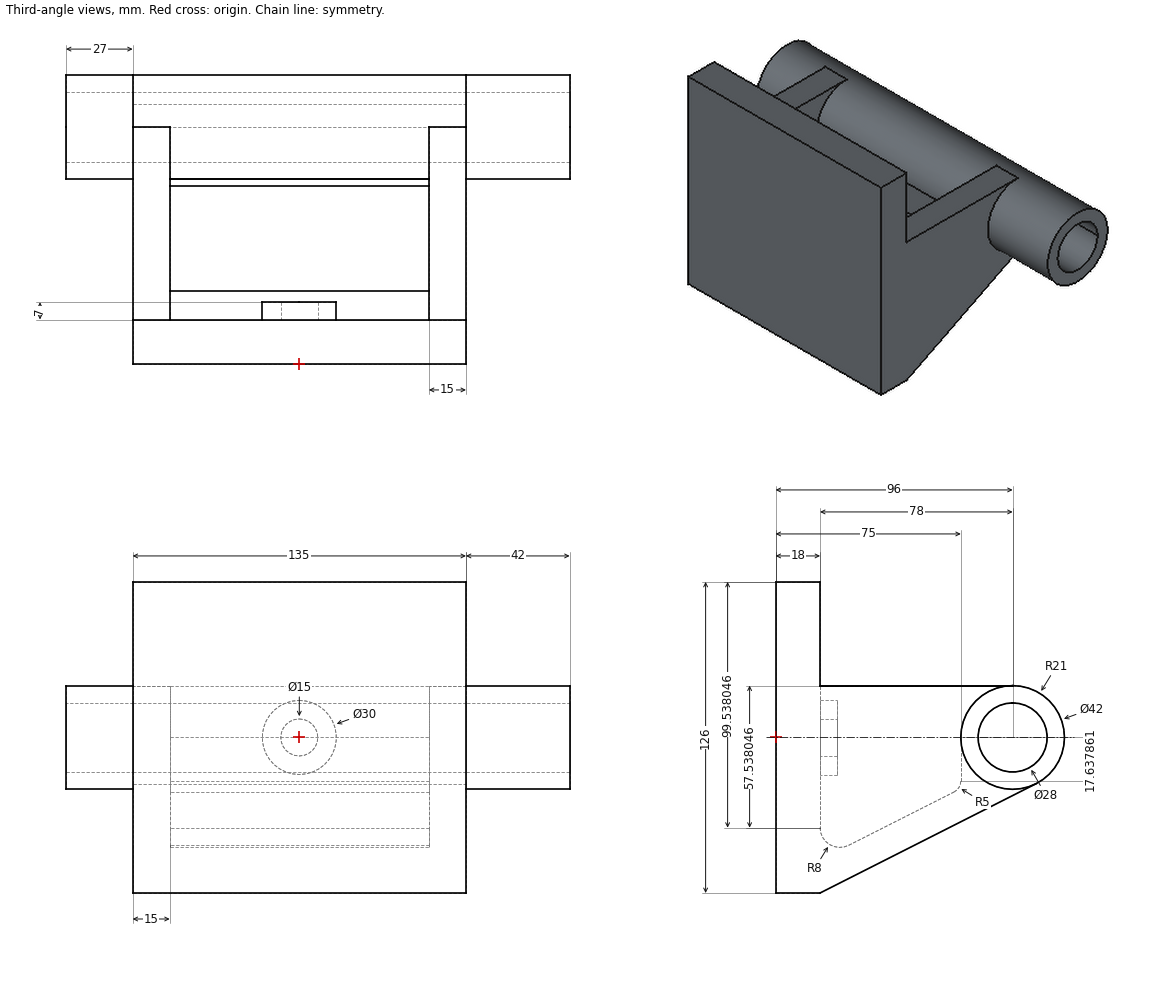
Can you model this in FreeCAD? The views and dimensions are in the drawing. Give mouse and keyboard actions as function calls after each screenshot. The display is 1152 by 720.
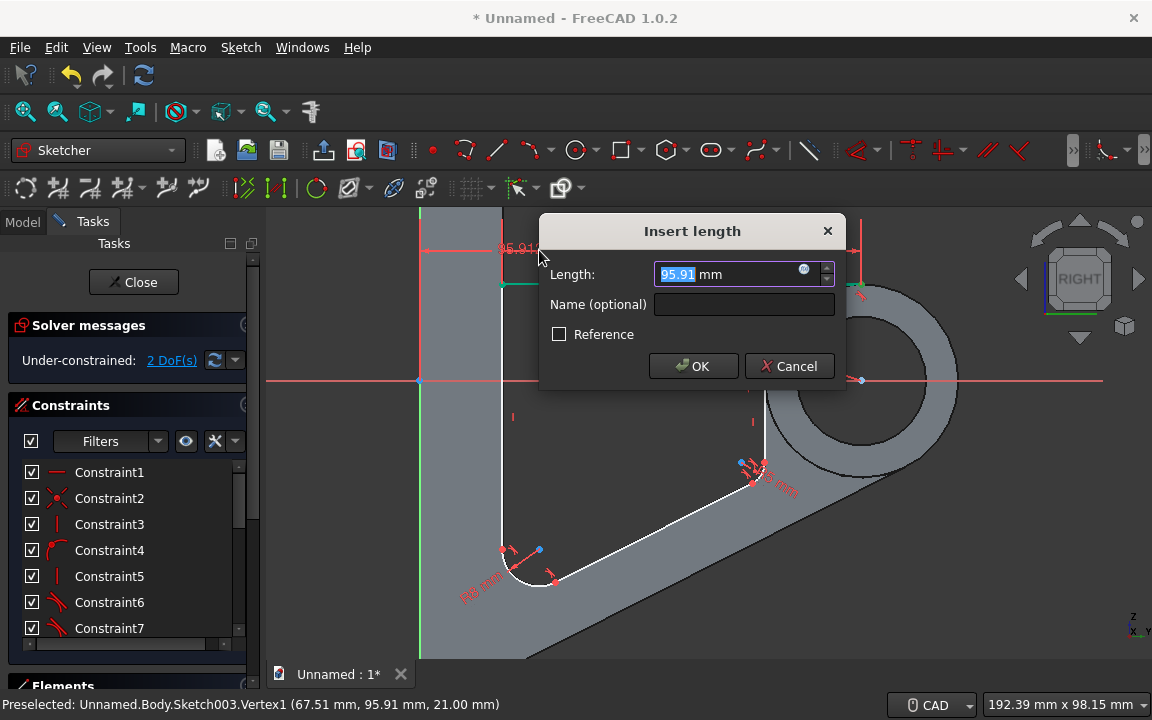
text(96)
key(Return)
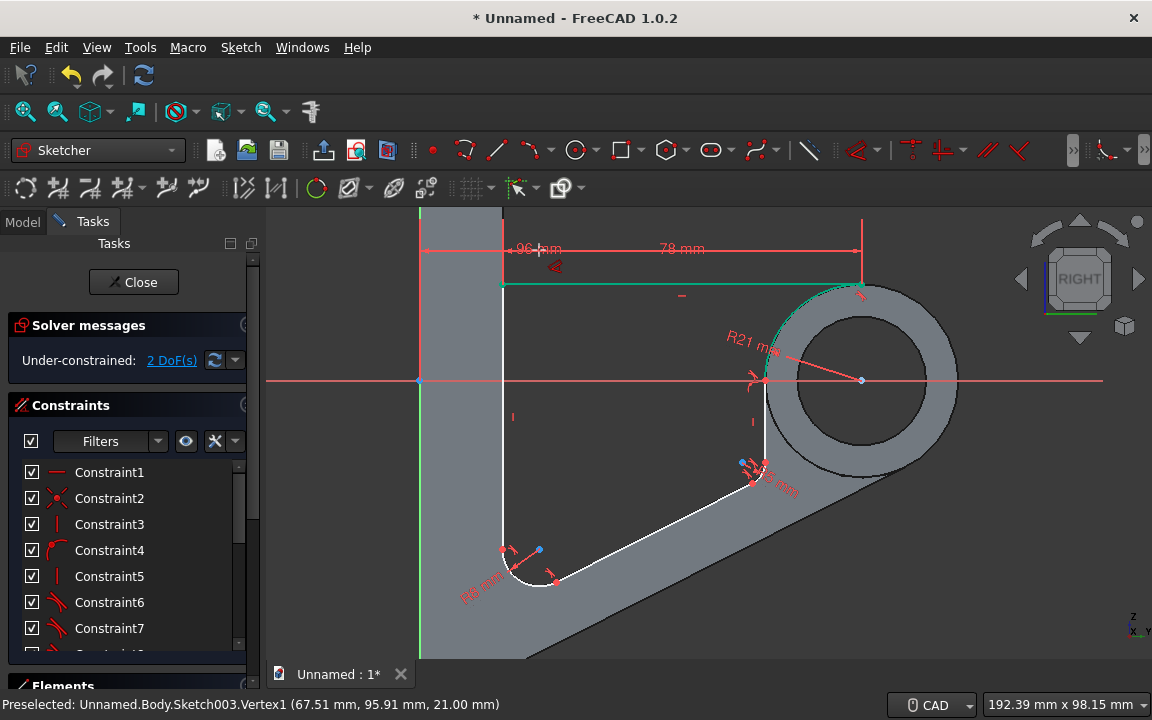
click(503, 364)
click(469, 417)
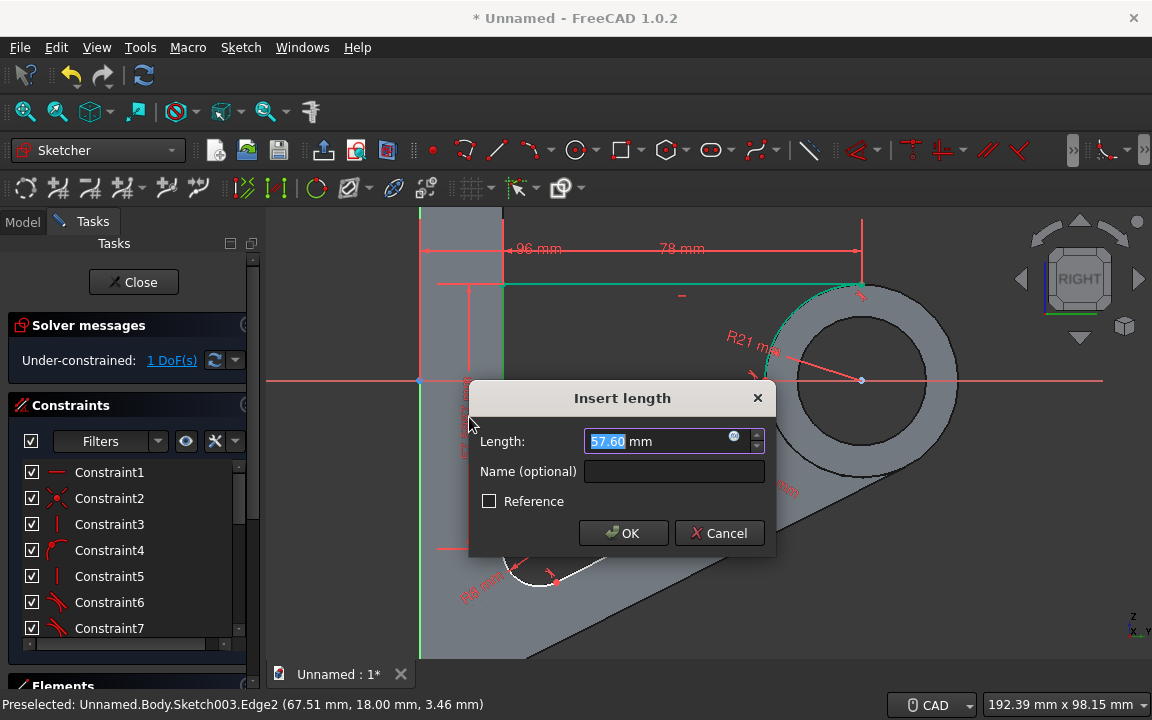
text(57.538046)
key(Return)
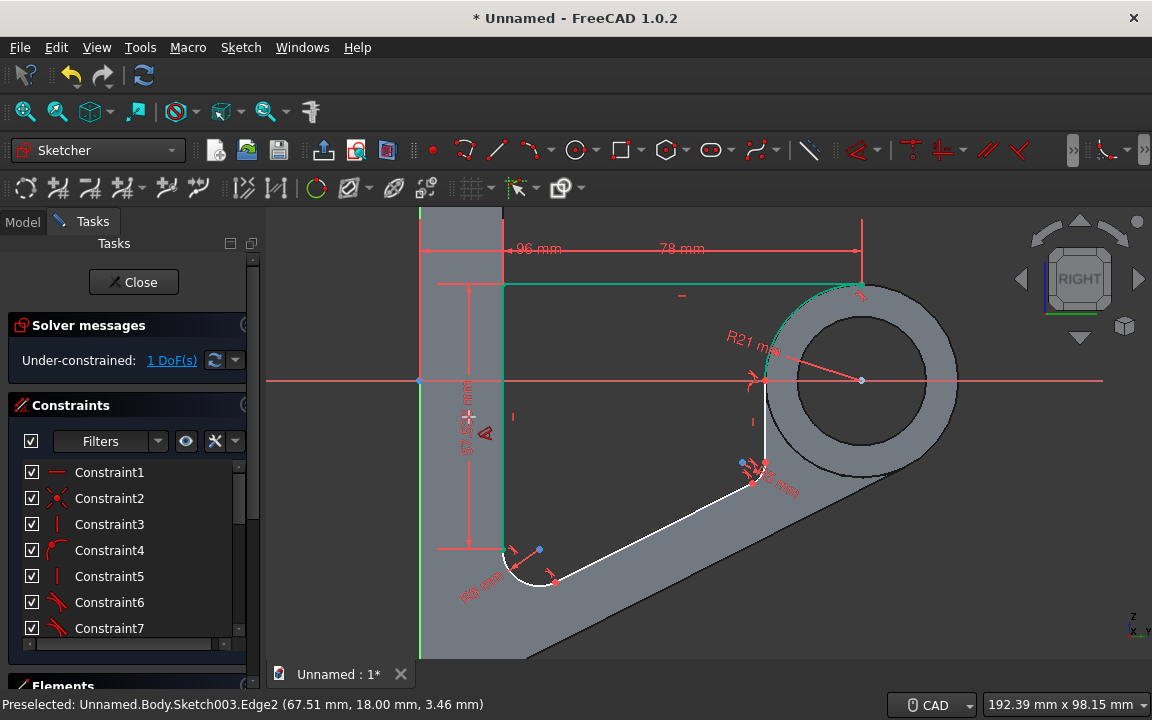
click(765, 438)
click(799, 422)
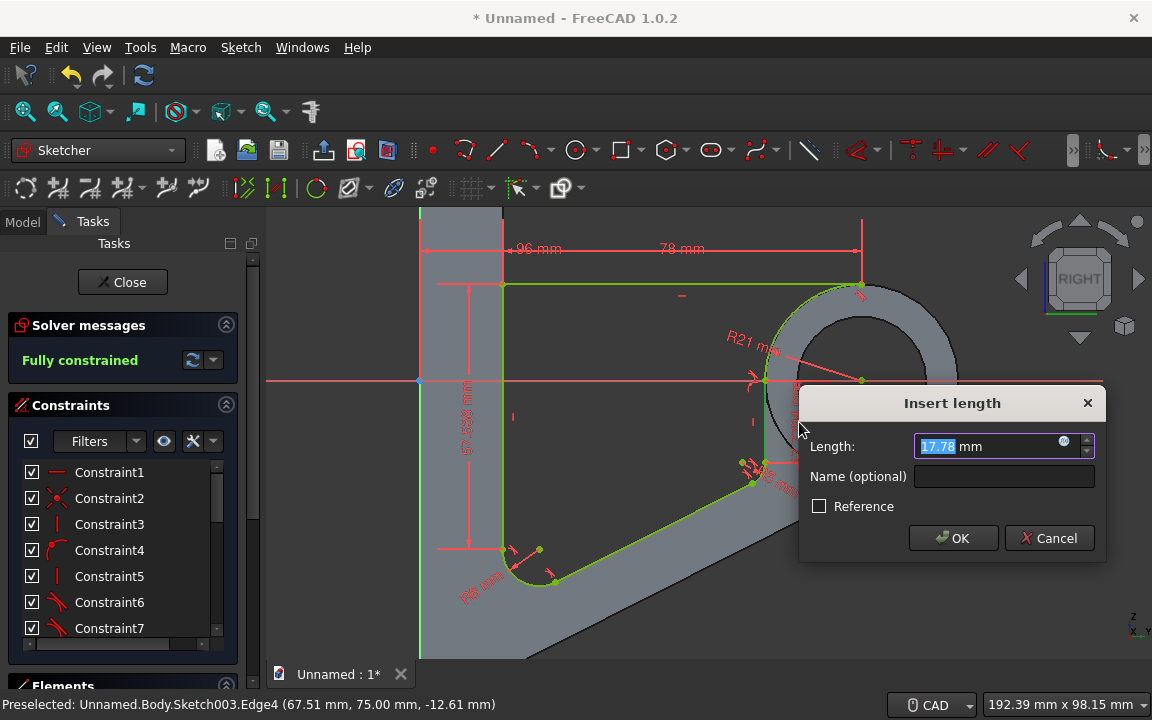
text(17.637861)
key(Return)
key(Escape)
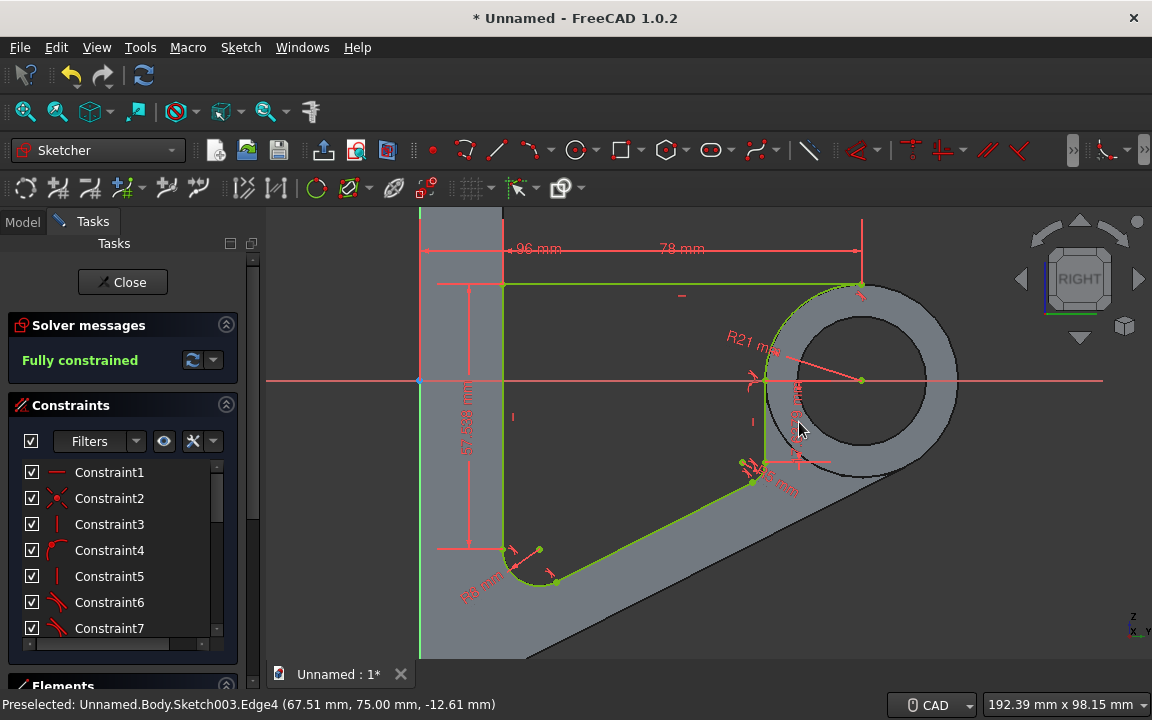
click(123, 282)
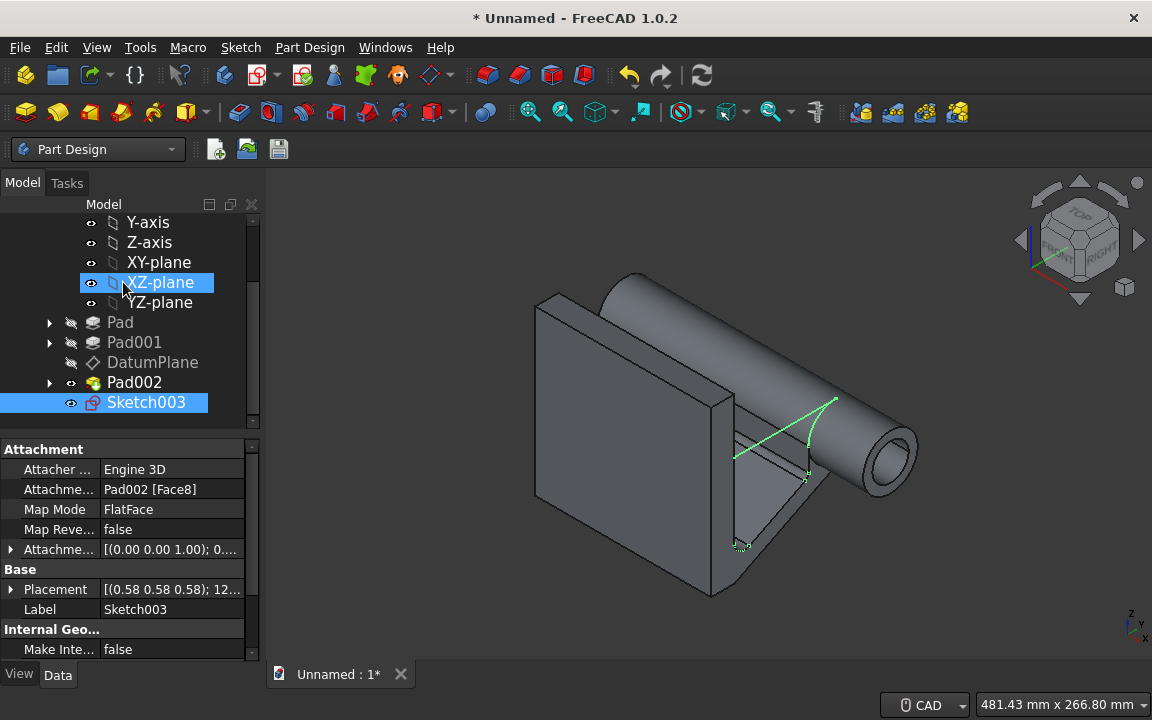
click(26, 112)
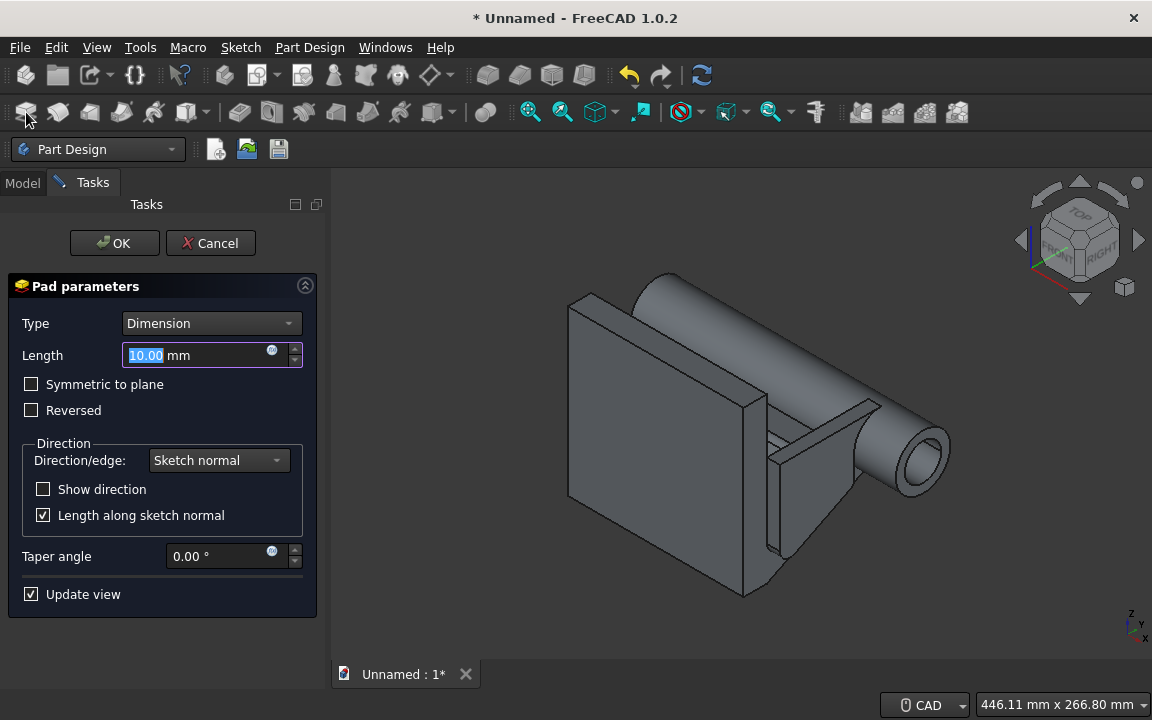
text(15)
key(Tab)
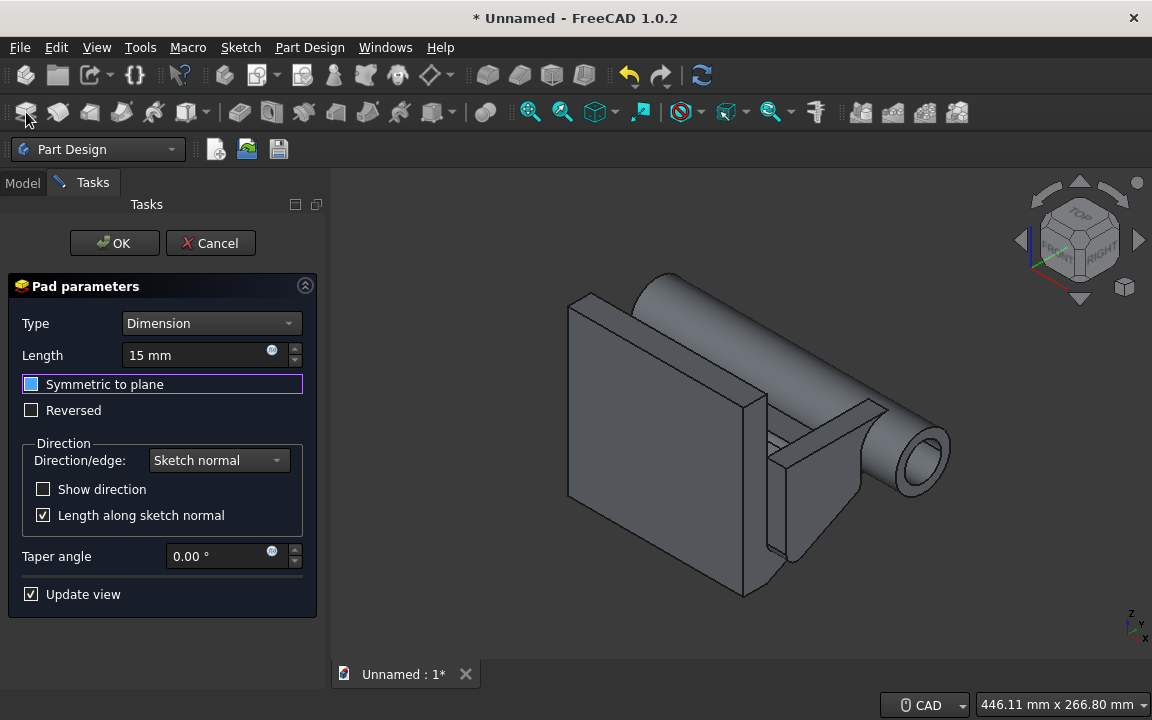
click(30, 410)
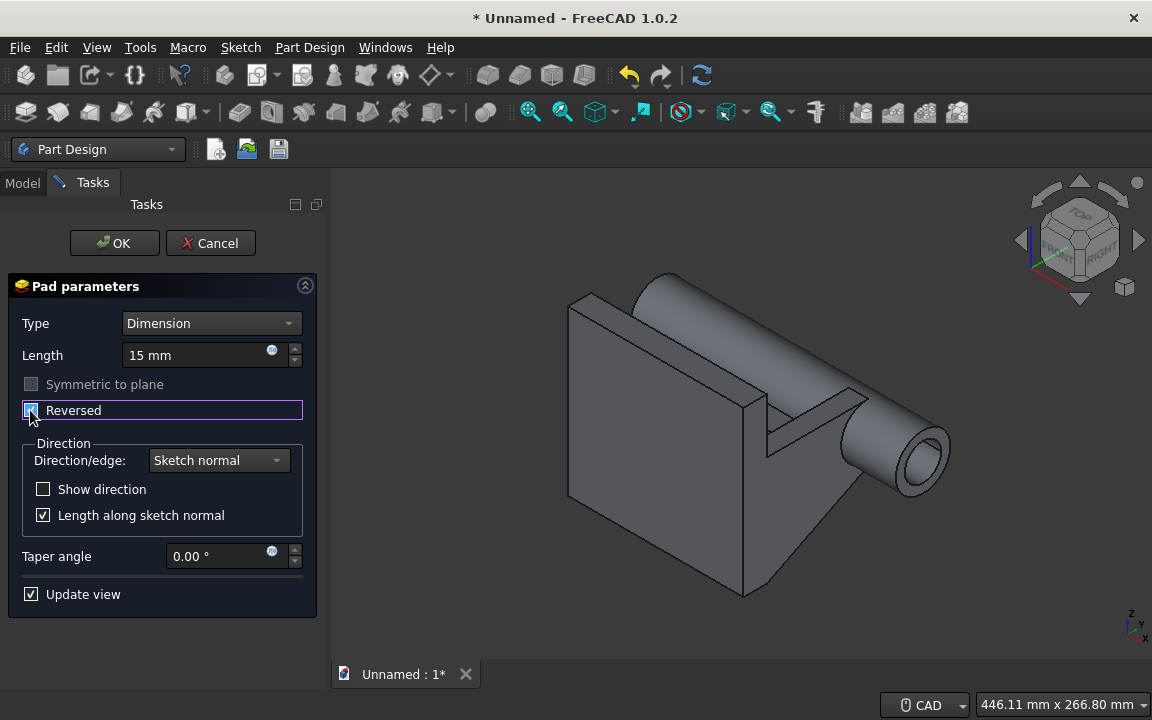
click(115, 243)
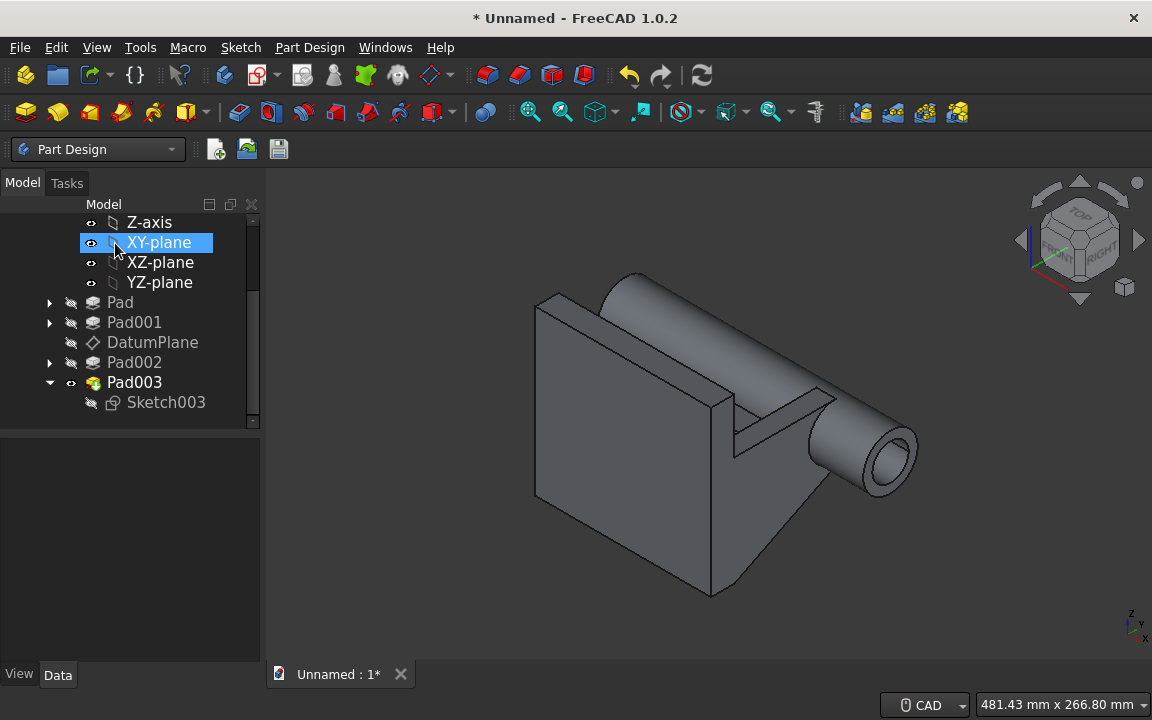
scroll(160, 318, down, 3)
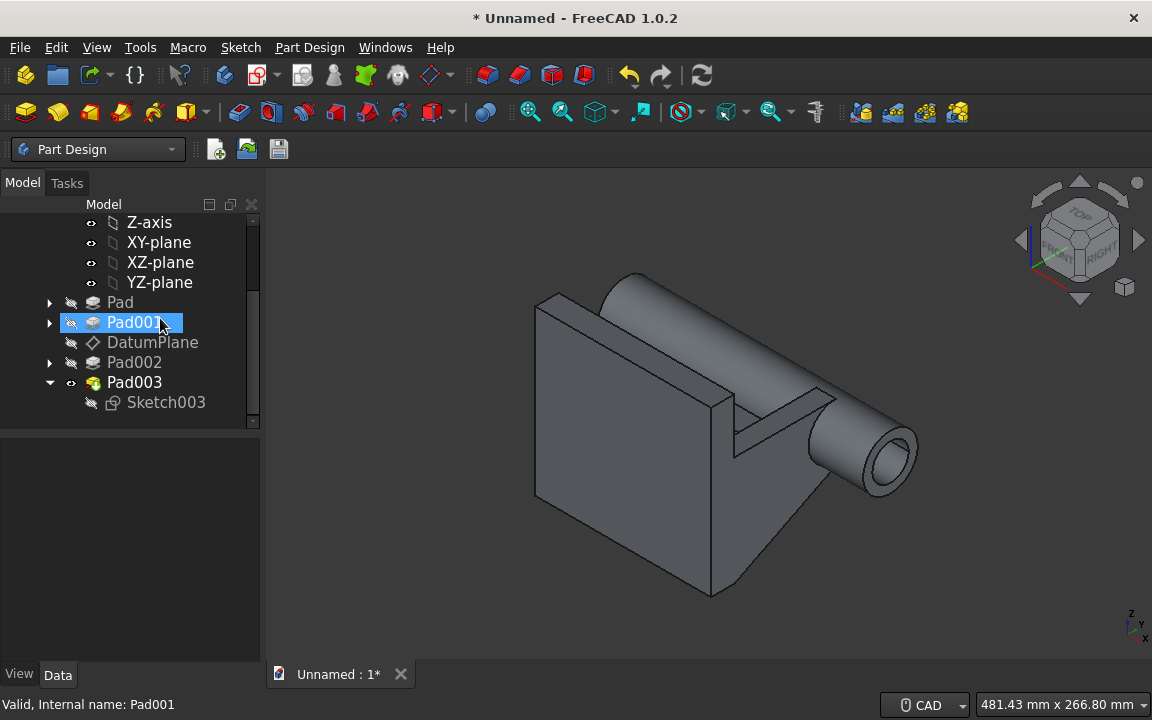
scroll(160, 318, up, 15)